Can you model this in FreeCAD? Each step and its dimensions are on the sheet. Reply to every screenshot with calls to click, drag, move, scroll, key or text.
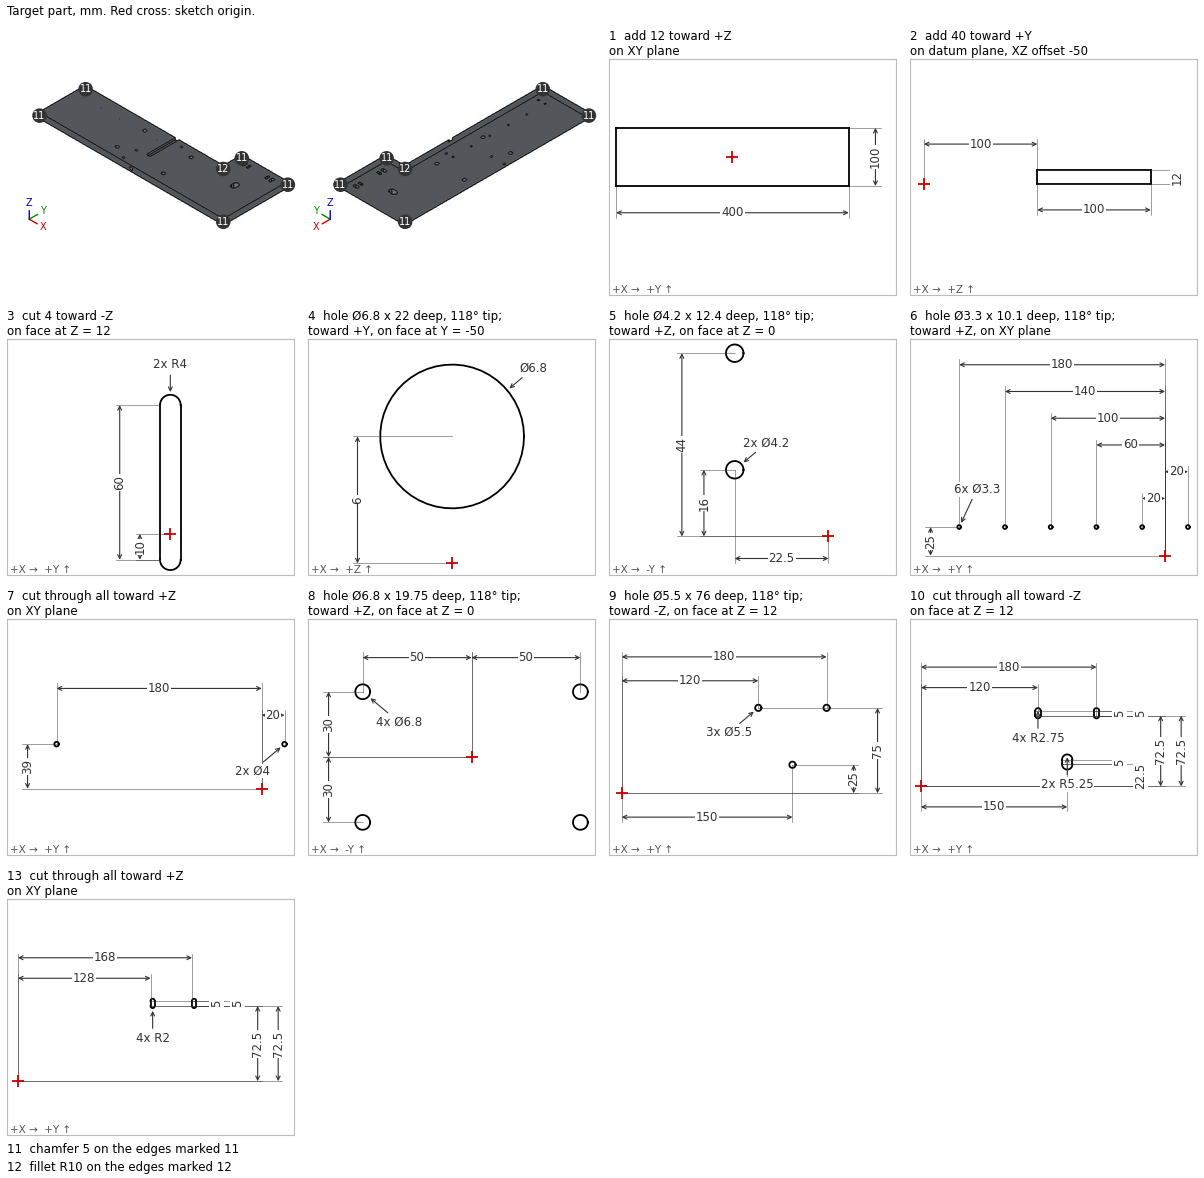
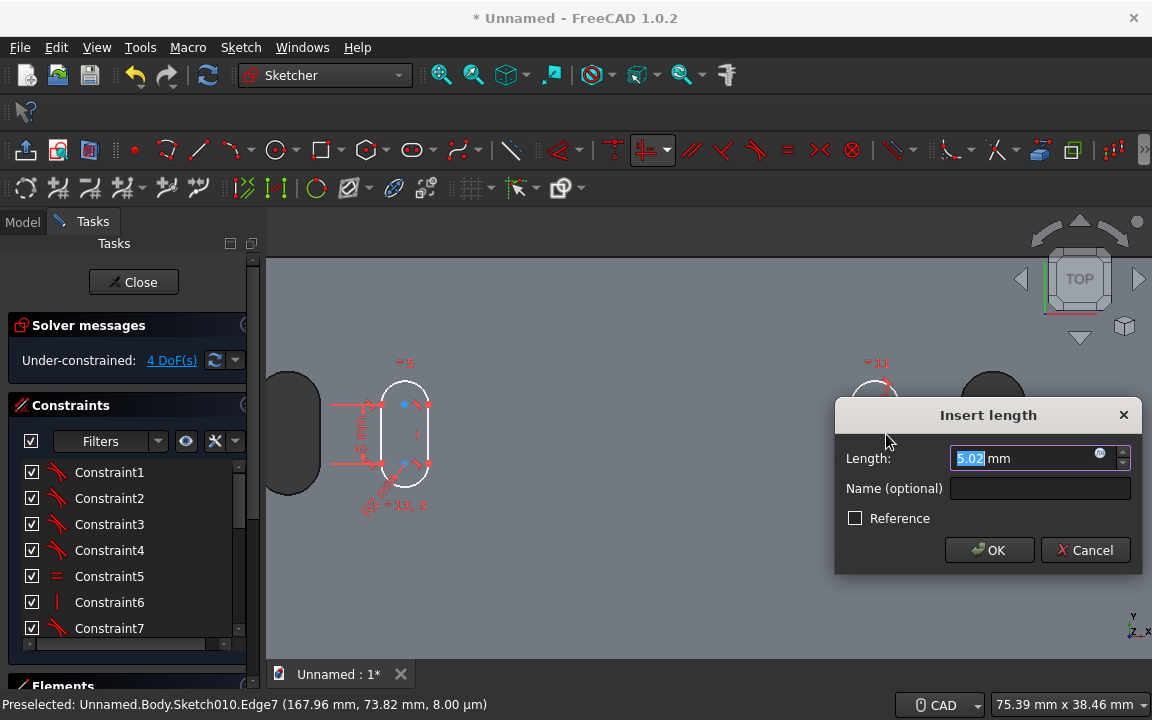
text(5)
key(Return)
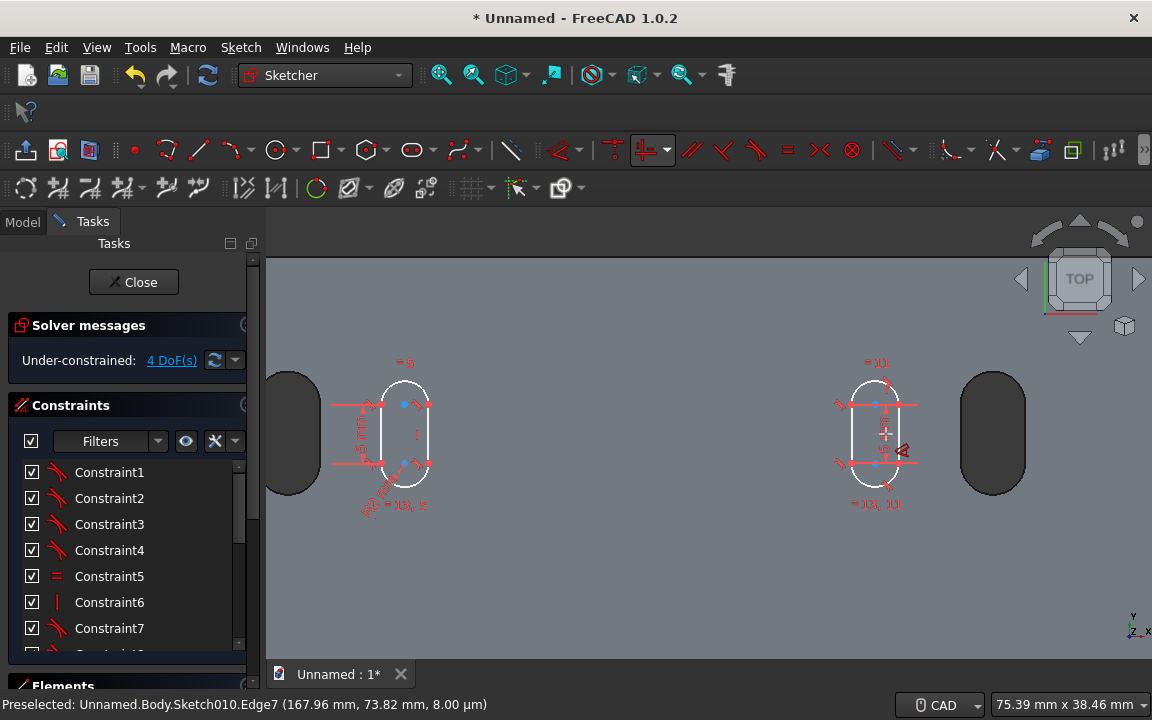
click(381, 464)
click(338, 406)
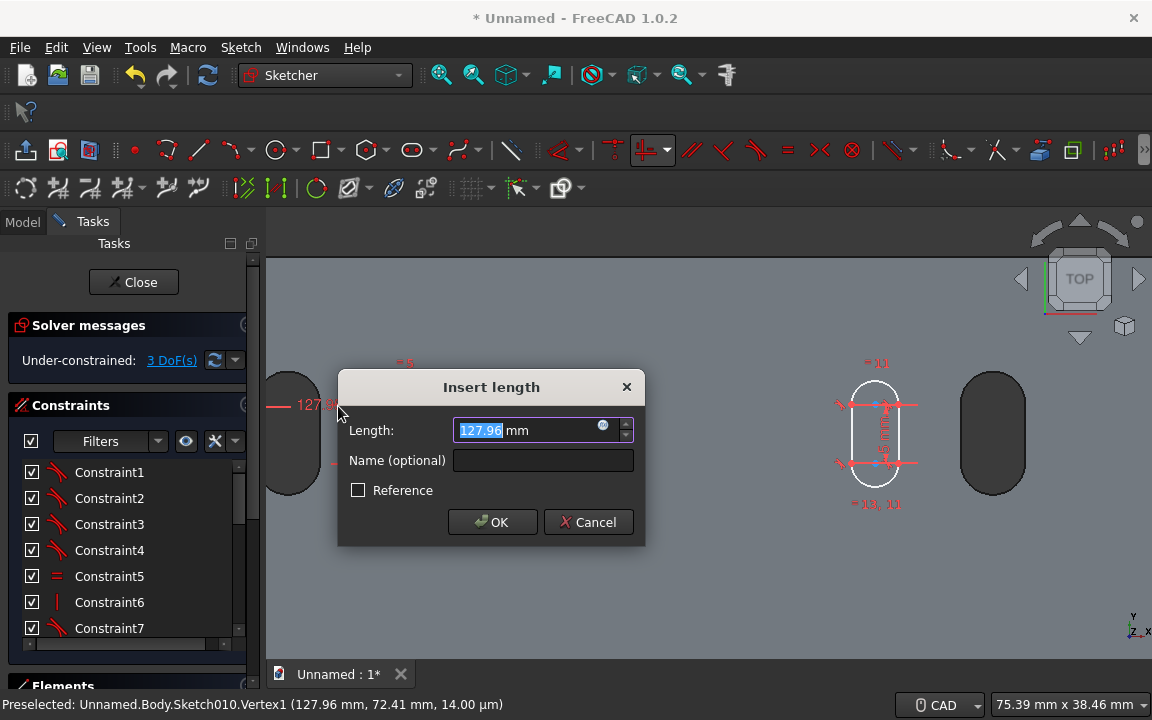
text(128)
key(Return)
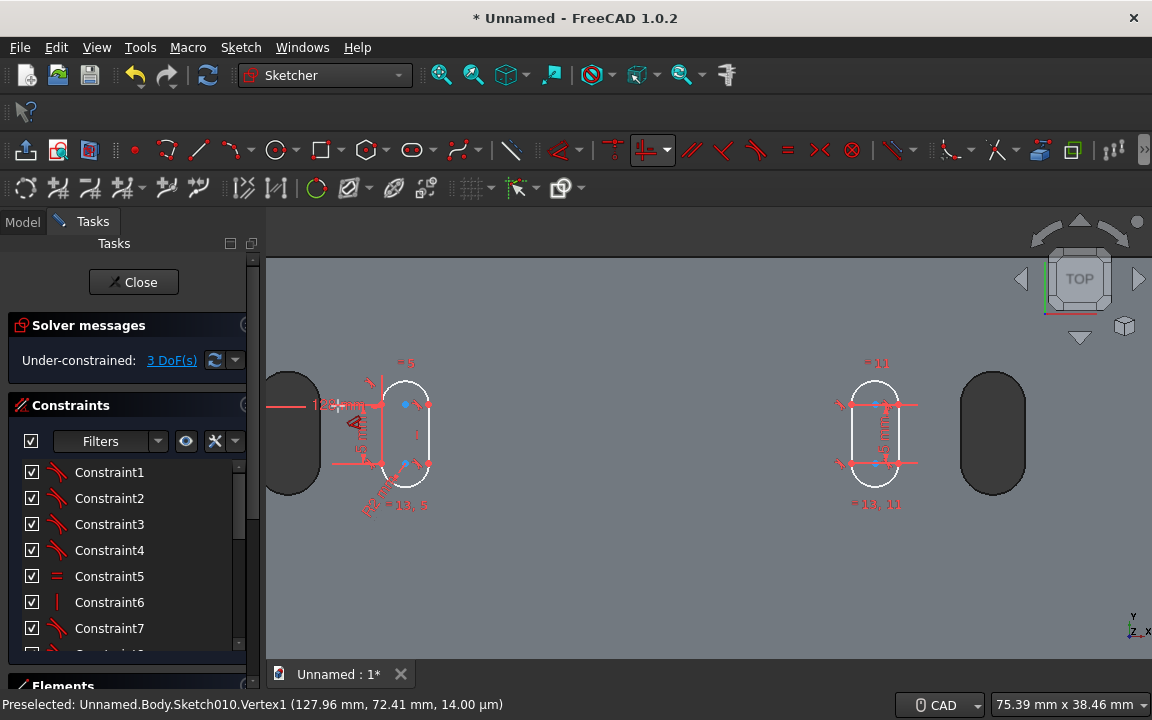
click(852, 463)
click(573, 429)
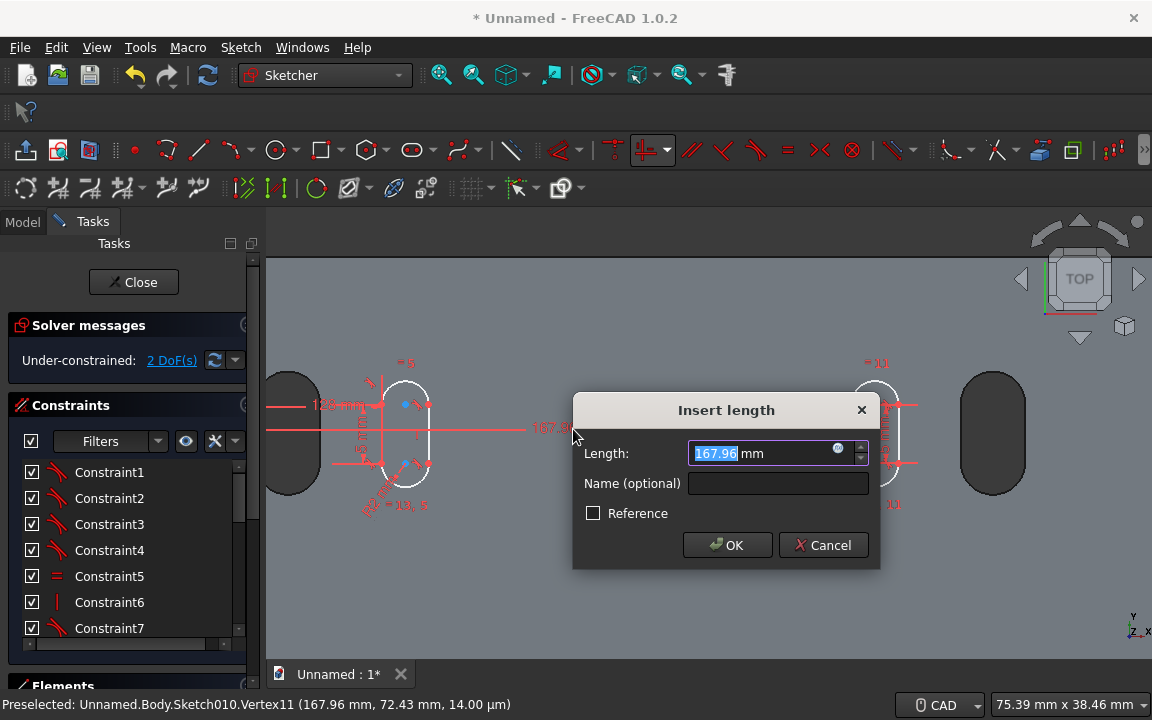
text(168)
key(Return)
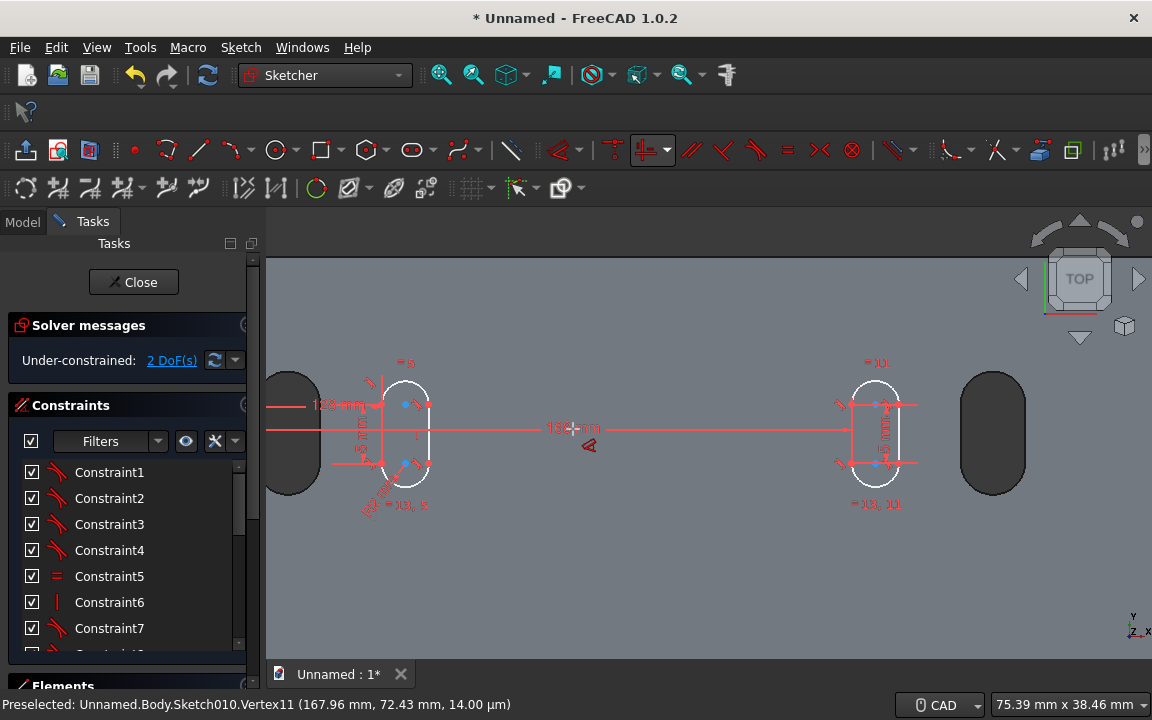
click(382, 464)
click(416, 547)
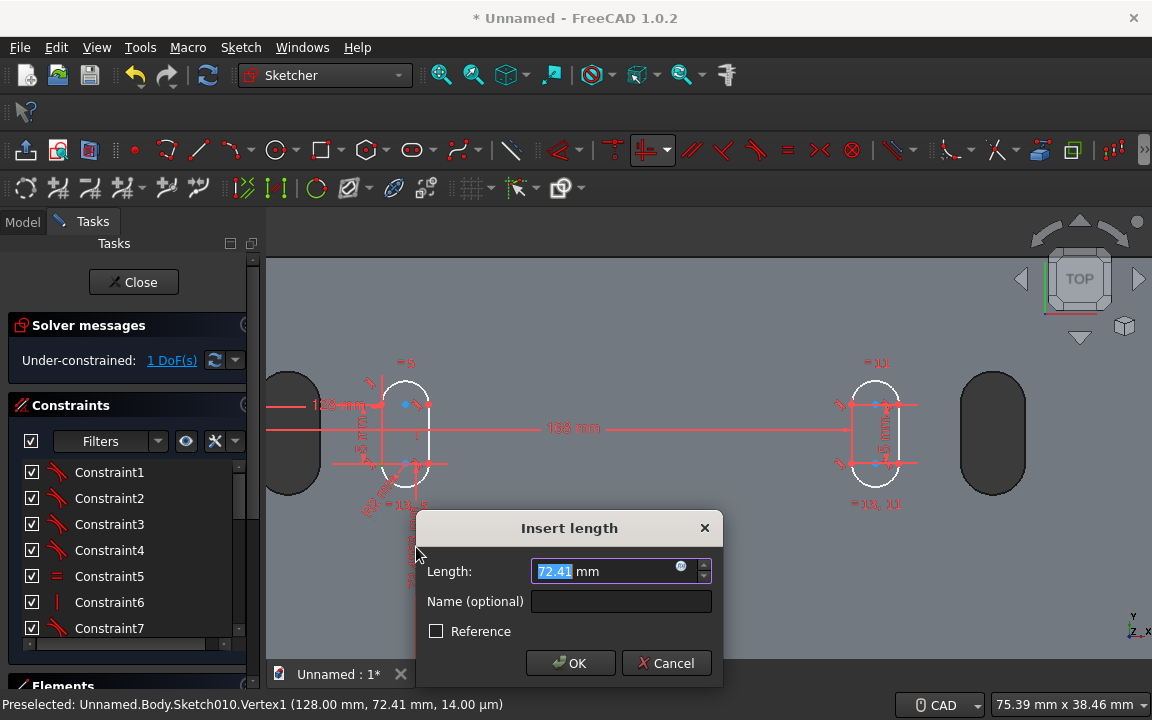
text(72.5)
key(Return)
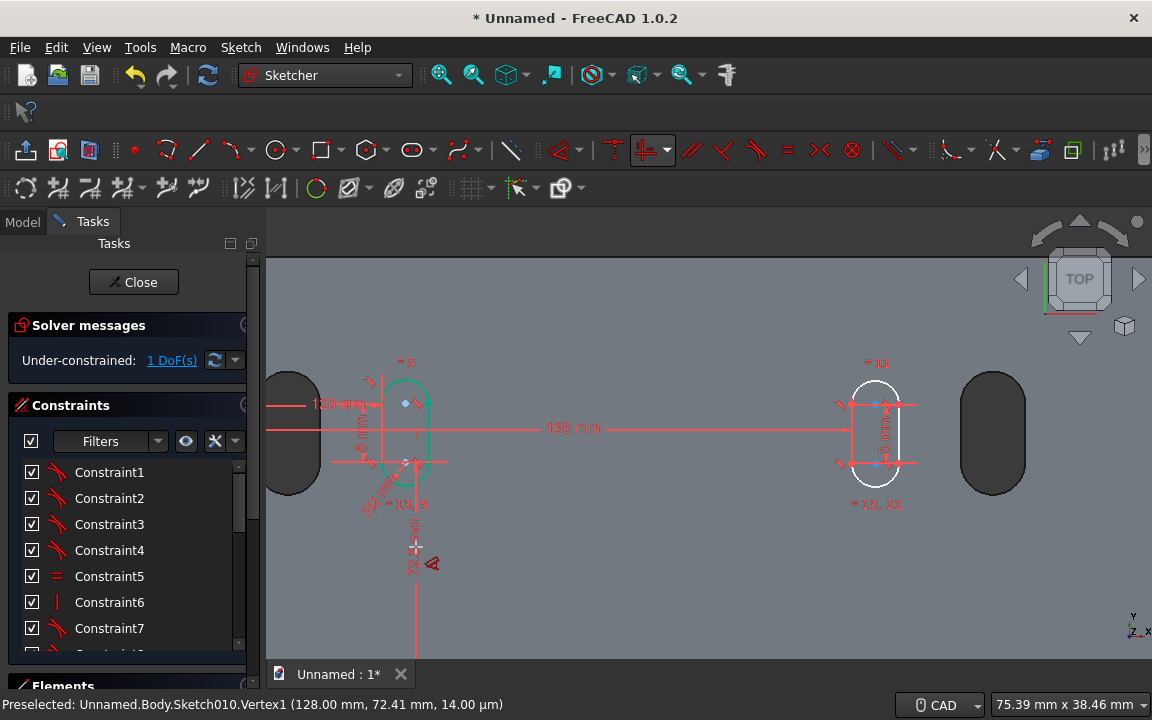
click(852, 463)
click(886, 547)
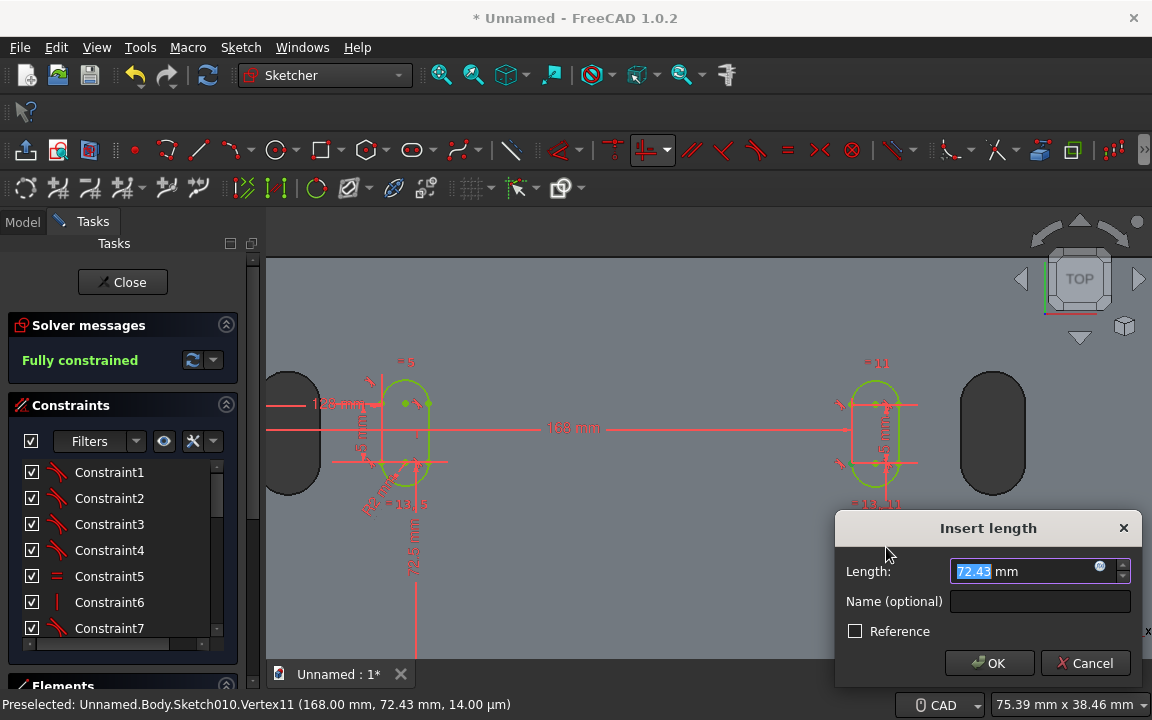
text(72.5)
key(Return)
key(Escape)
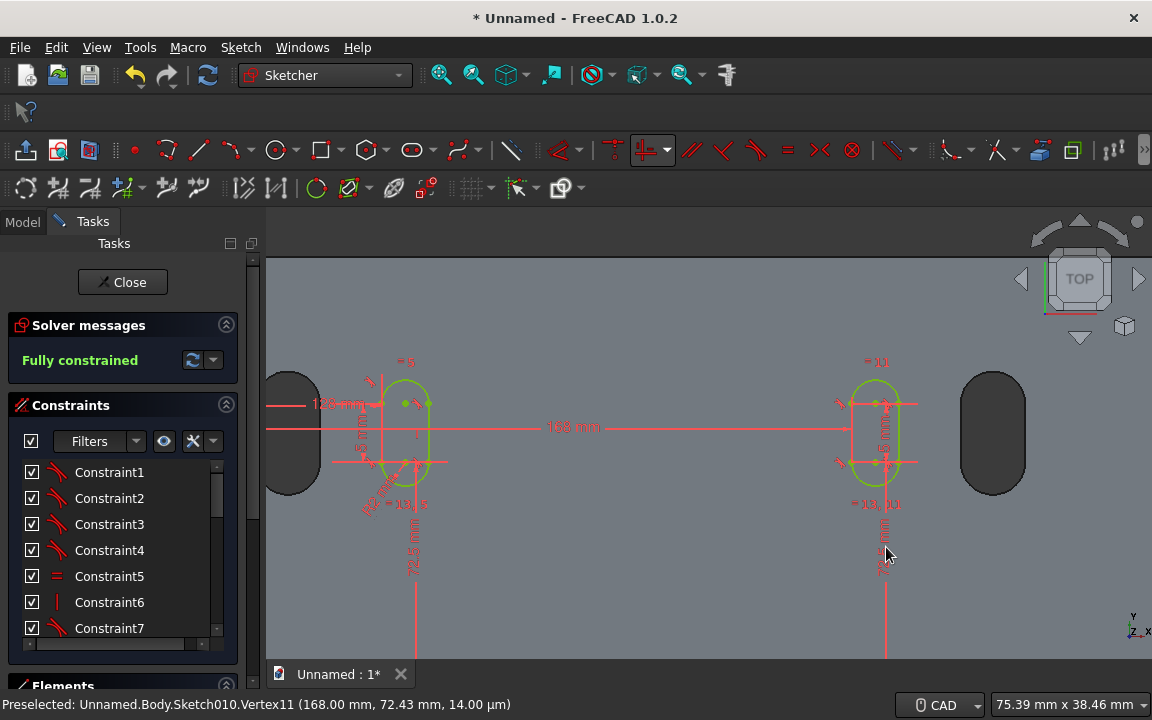
click(123, 282)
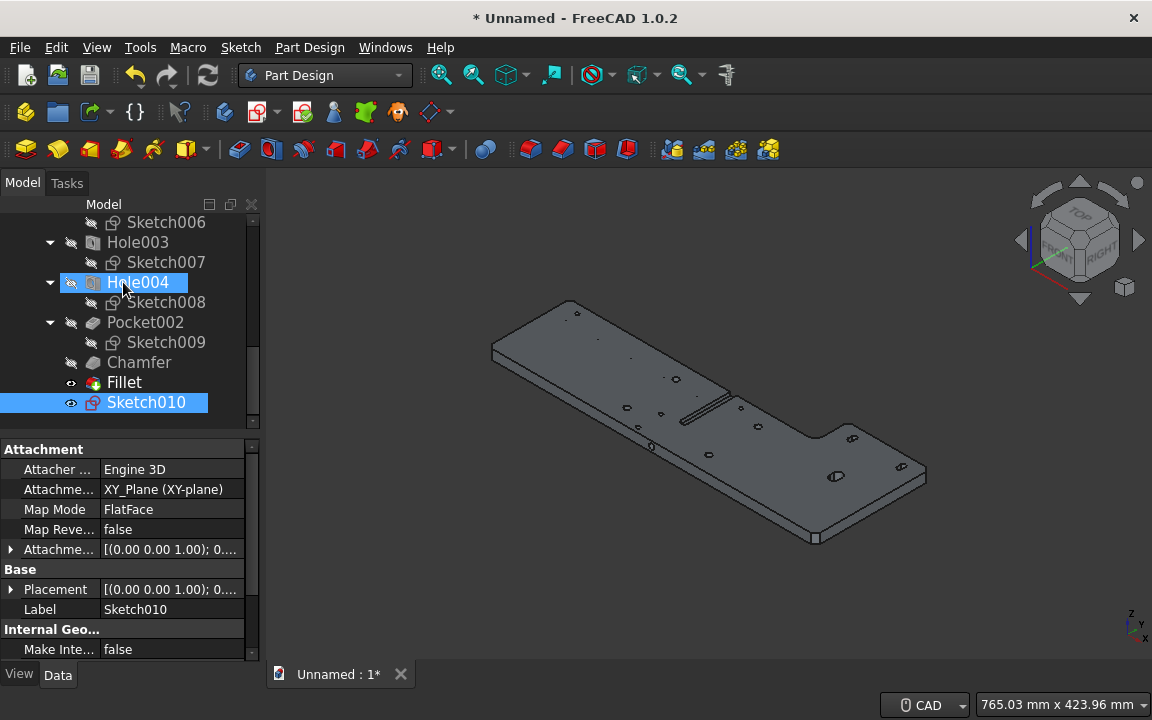
click(240, 150)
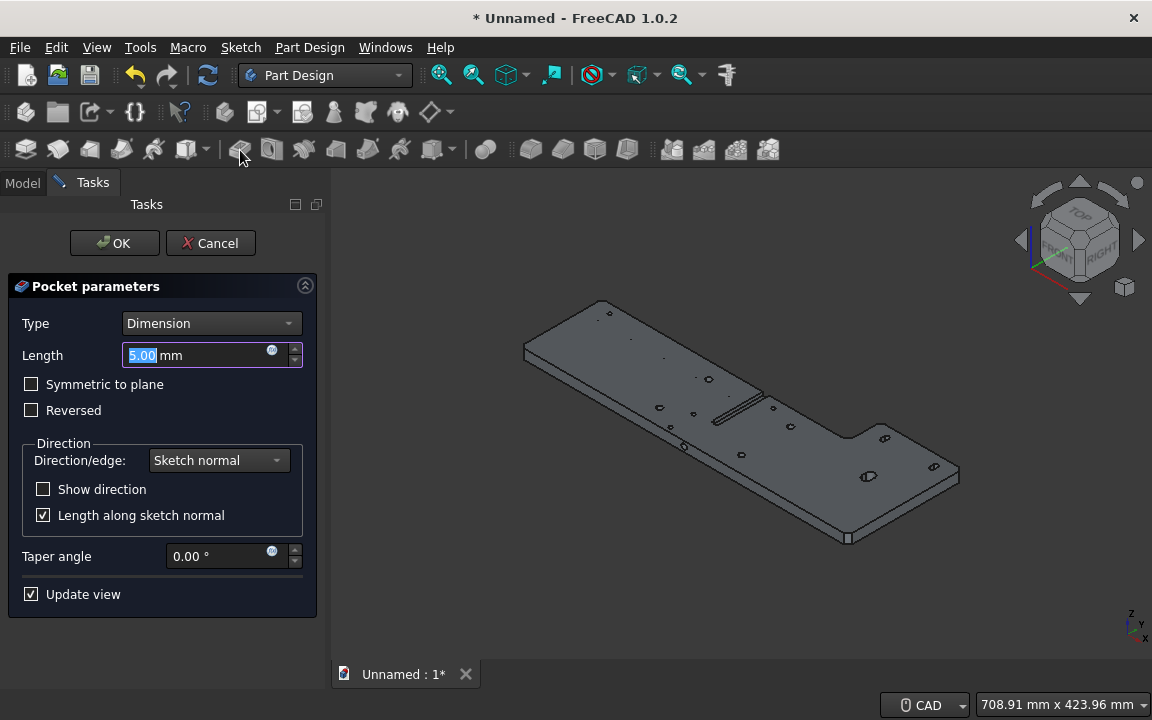
click(212, 324)